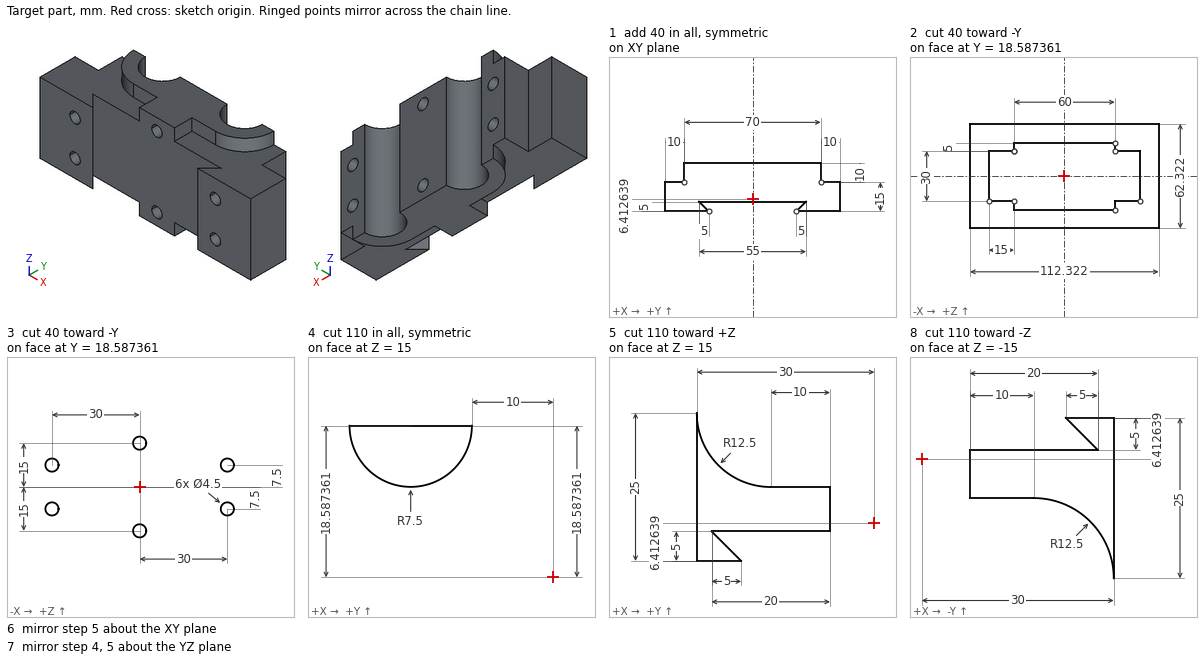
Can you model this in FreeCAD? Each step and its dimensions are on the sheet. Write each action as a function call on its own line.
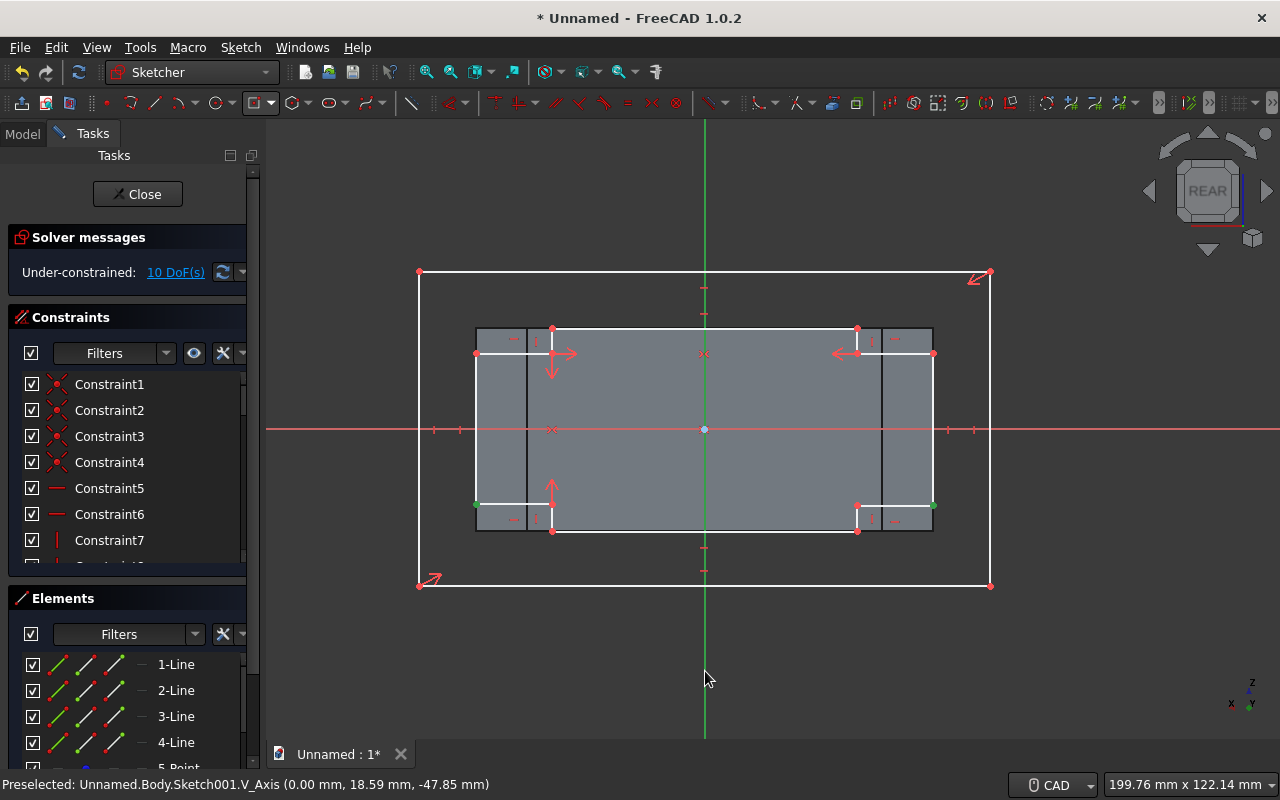
click(652, 104)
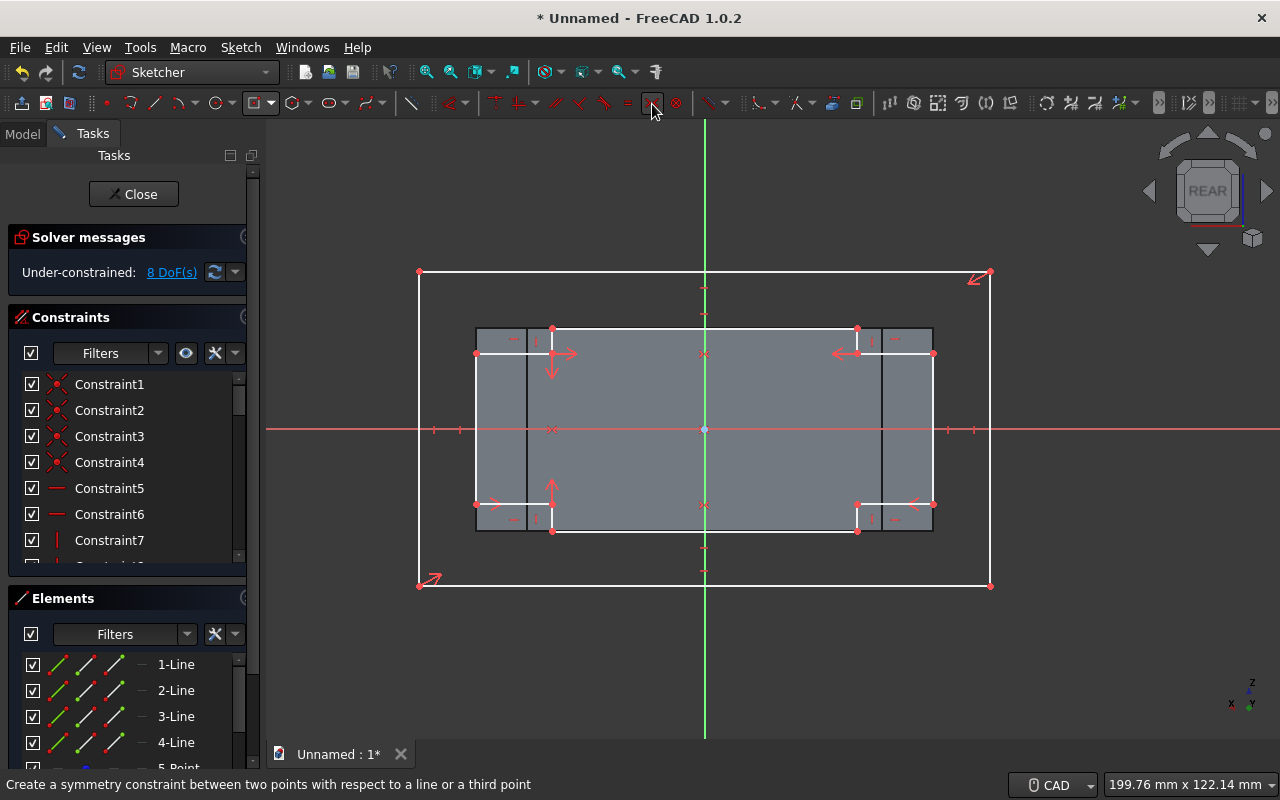
click(857, 329)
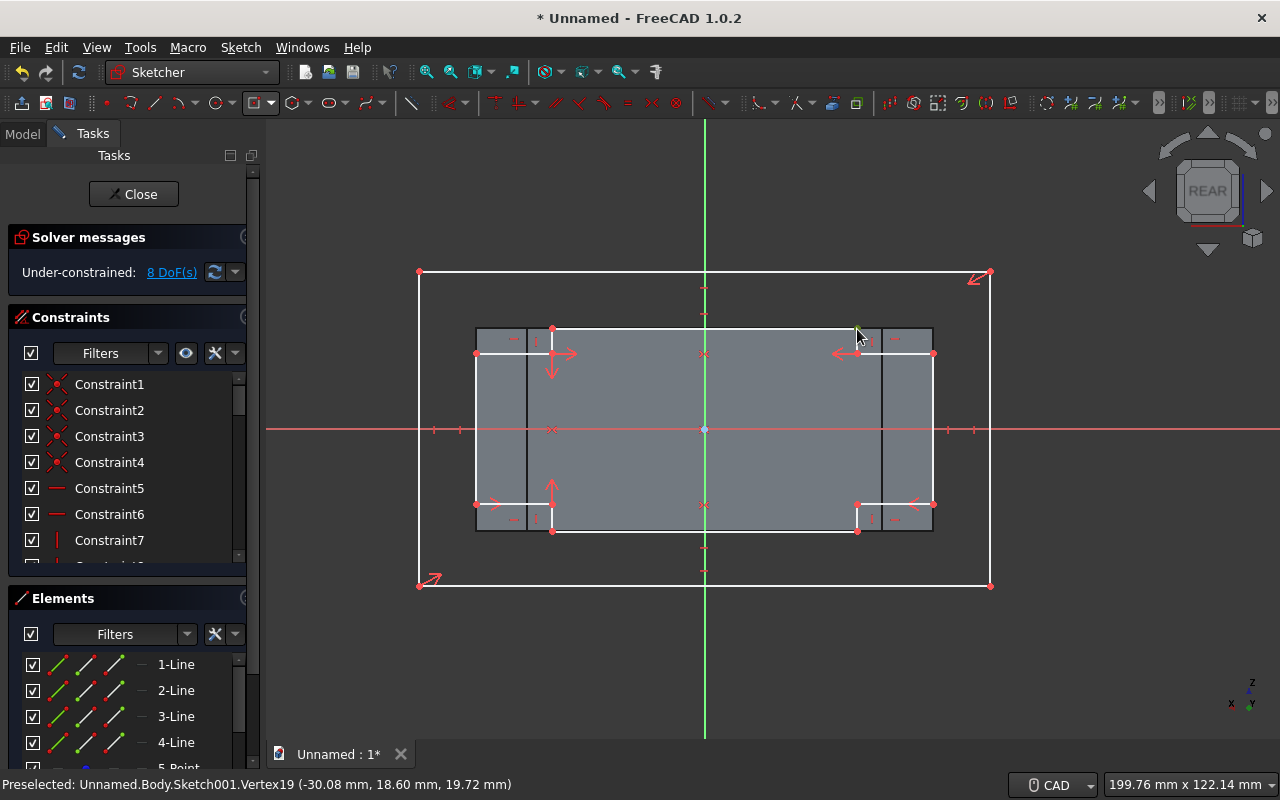
click(857, 532)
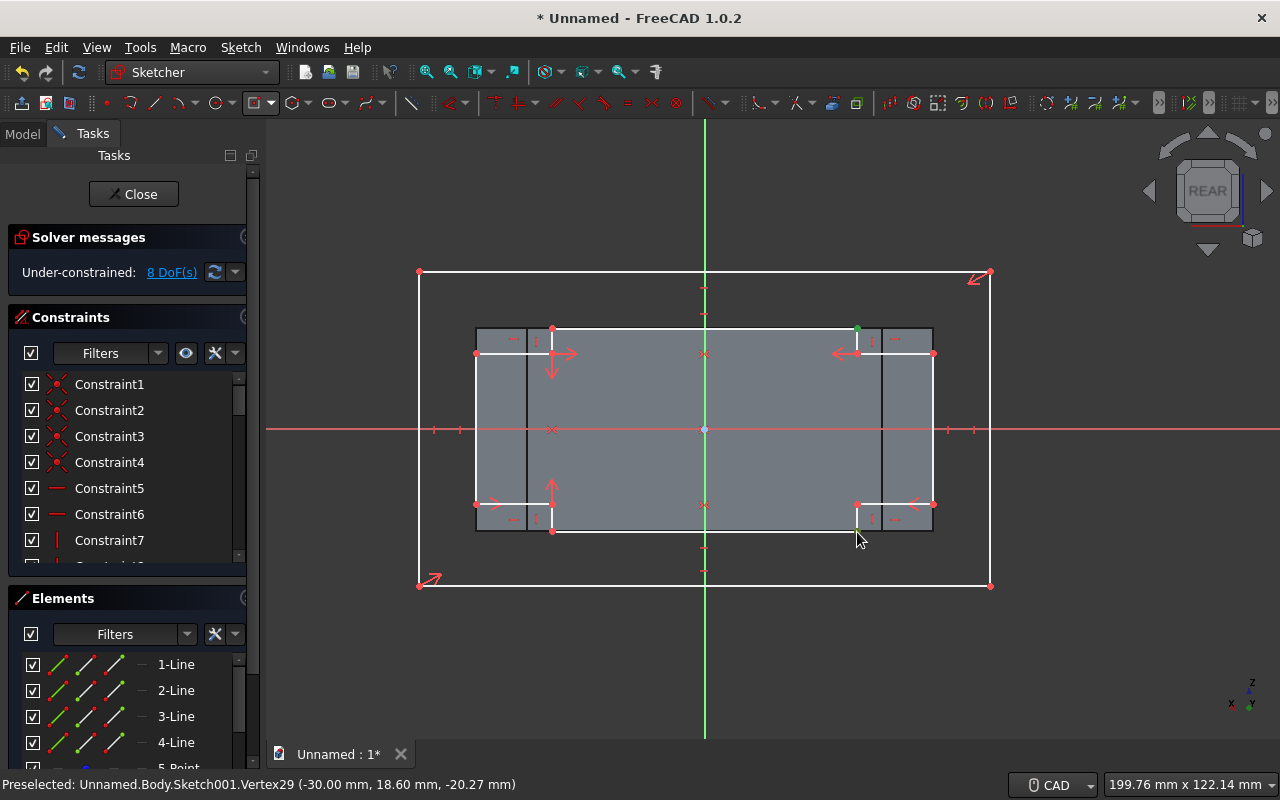
click(353, 429)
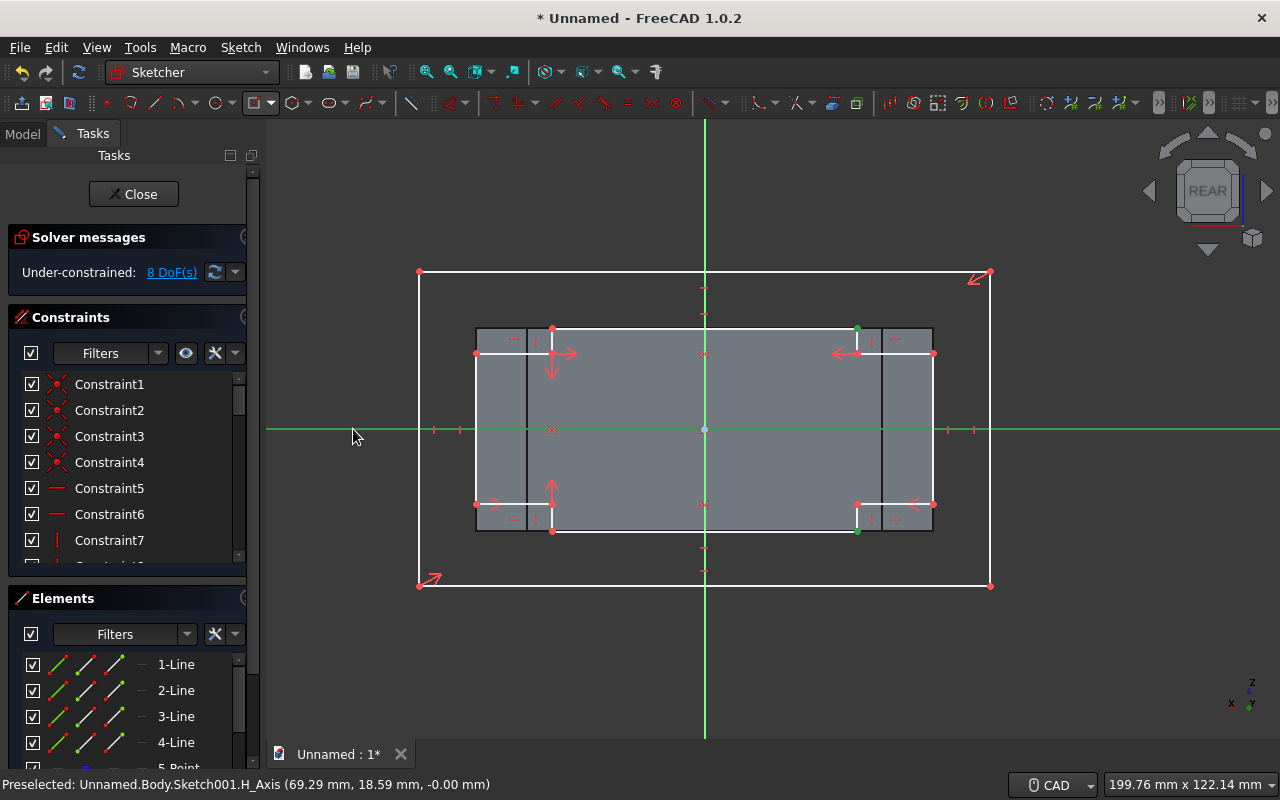
key(s)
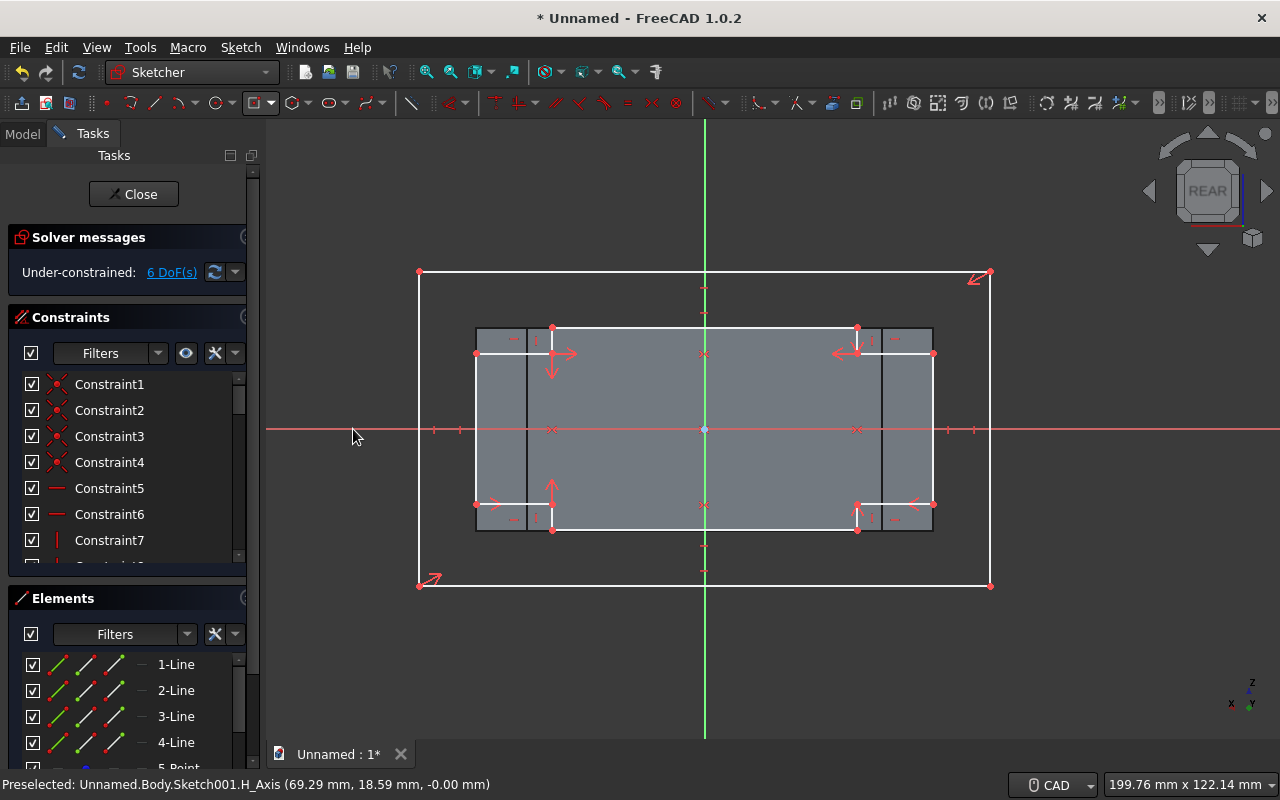
key(d)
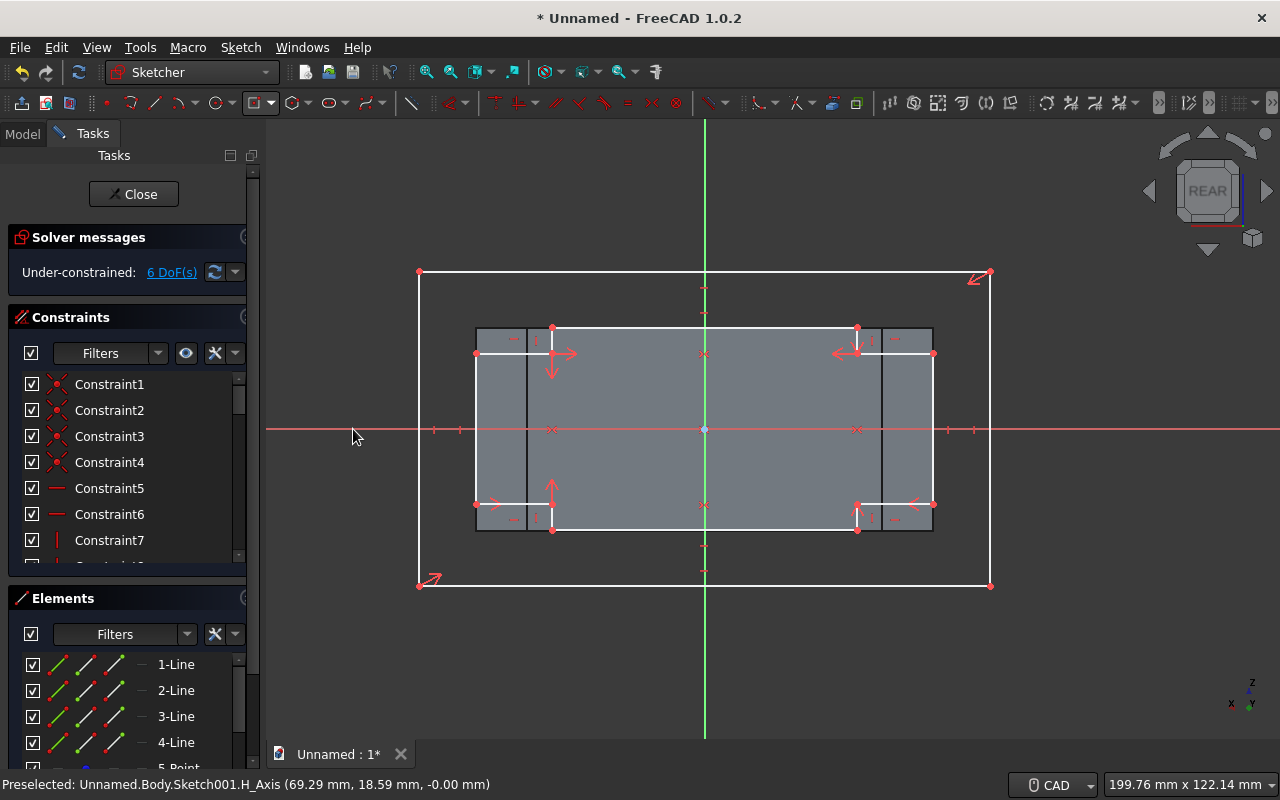
scroll(552, 343, up, 3)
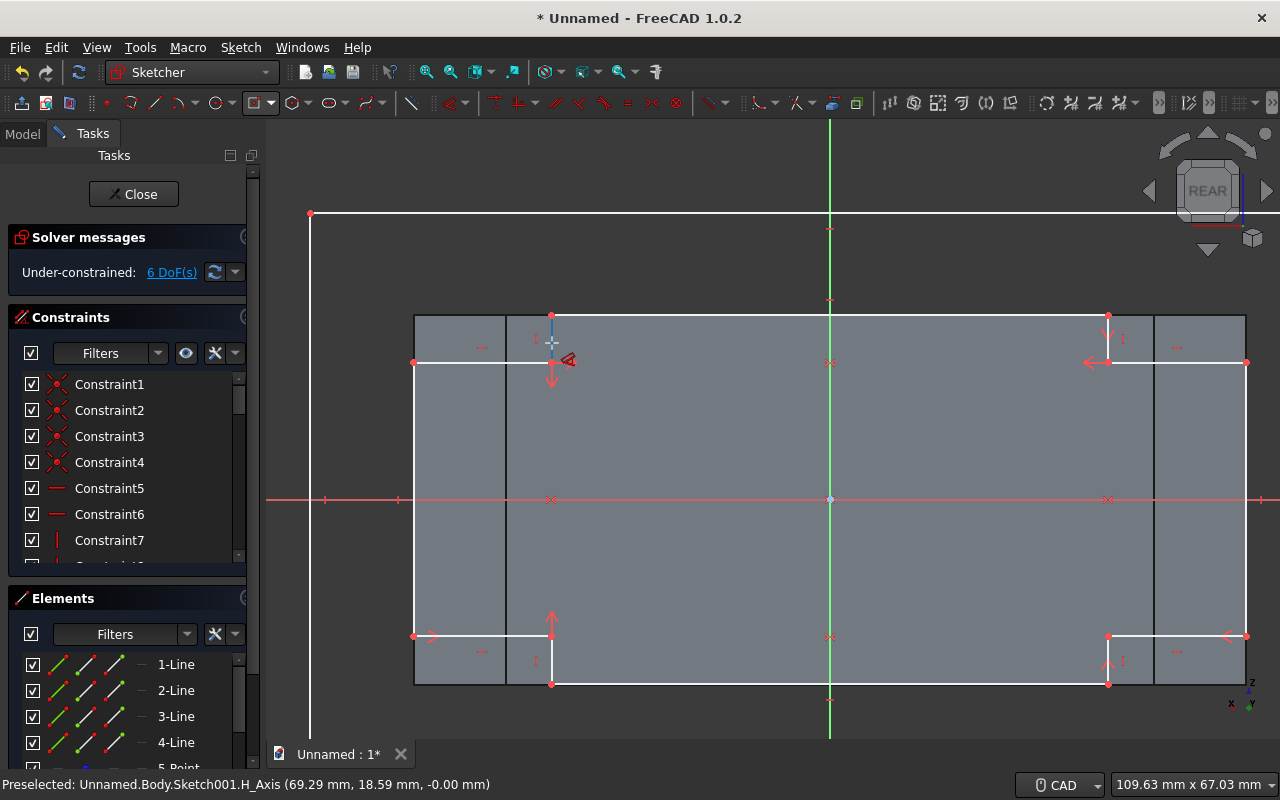
click(552, 344)
click(518, 339)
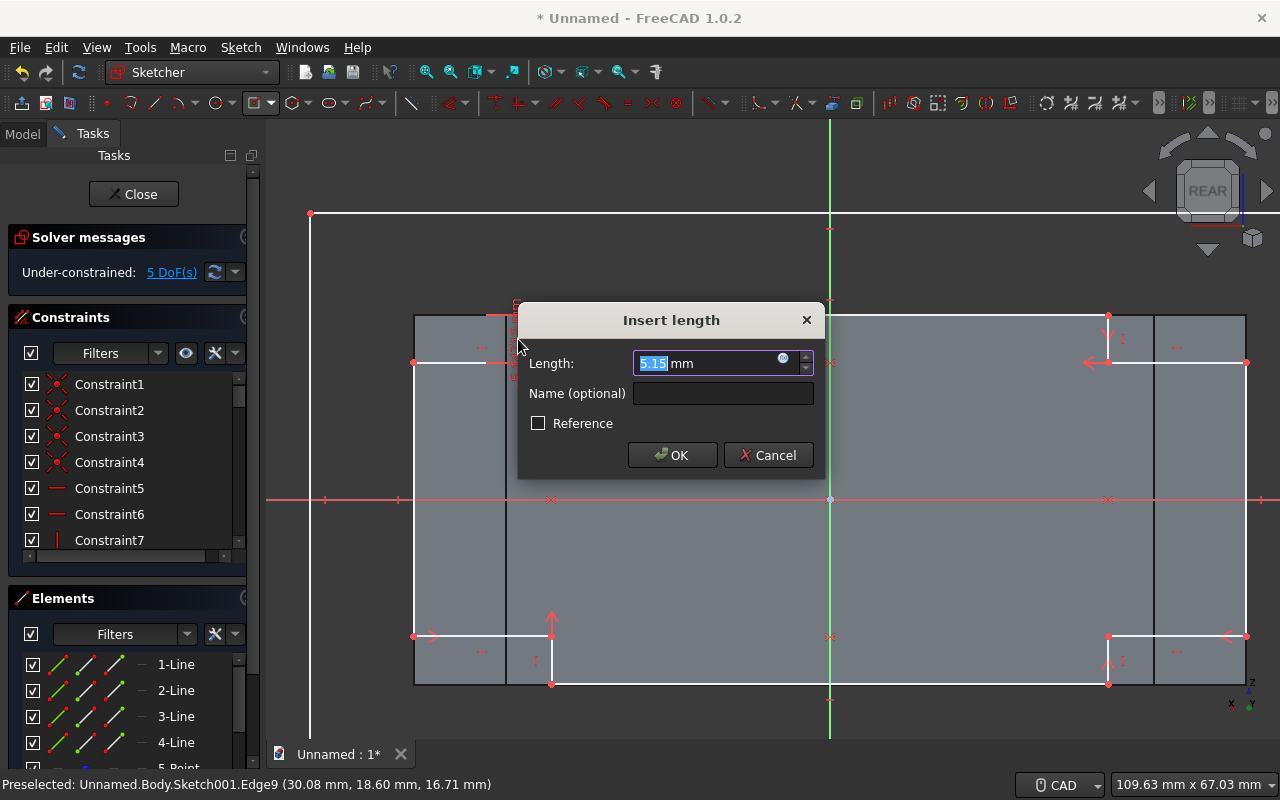
text(5)
key(Return)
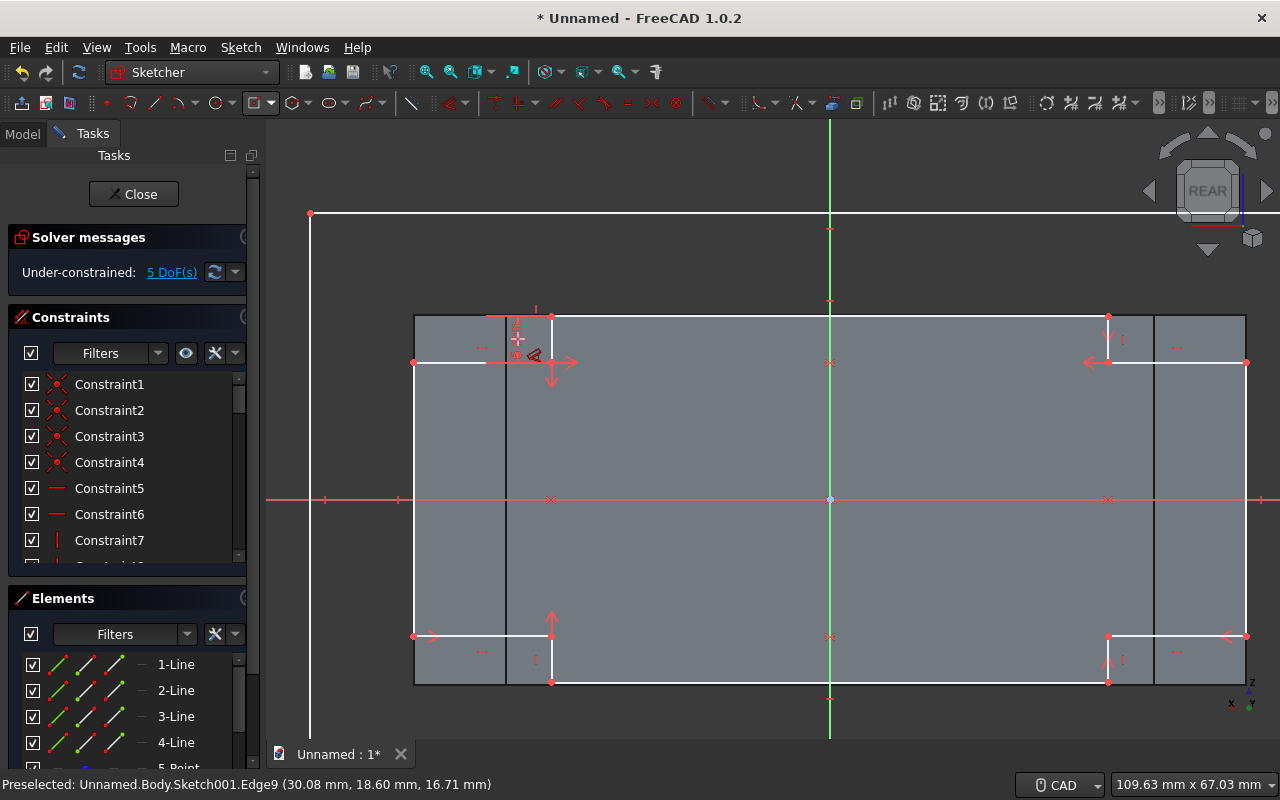
click(510, 636)
click(483, 670)